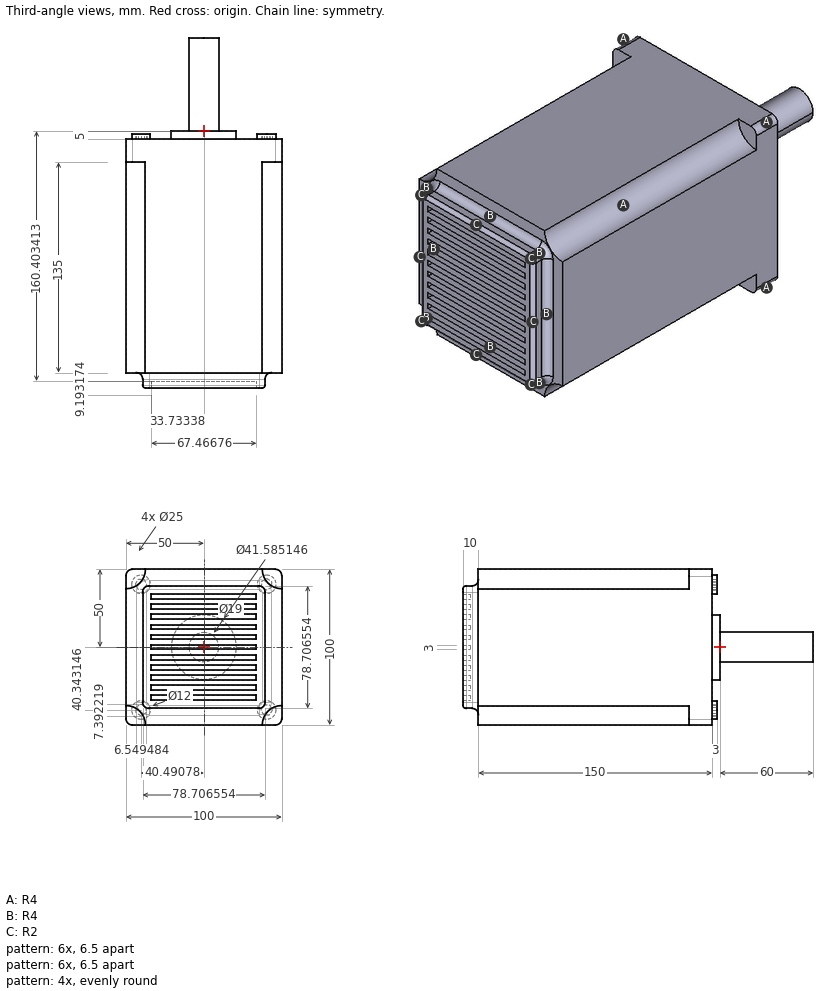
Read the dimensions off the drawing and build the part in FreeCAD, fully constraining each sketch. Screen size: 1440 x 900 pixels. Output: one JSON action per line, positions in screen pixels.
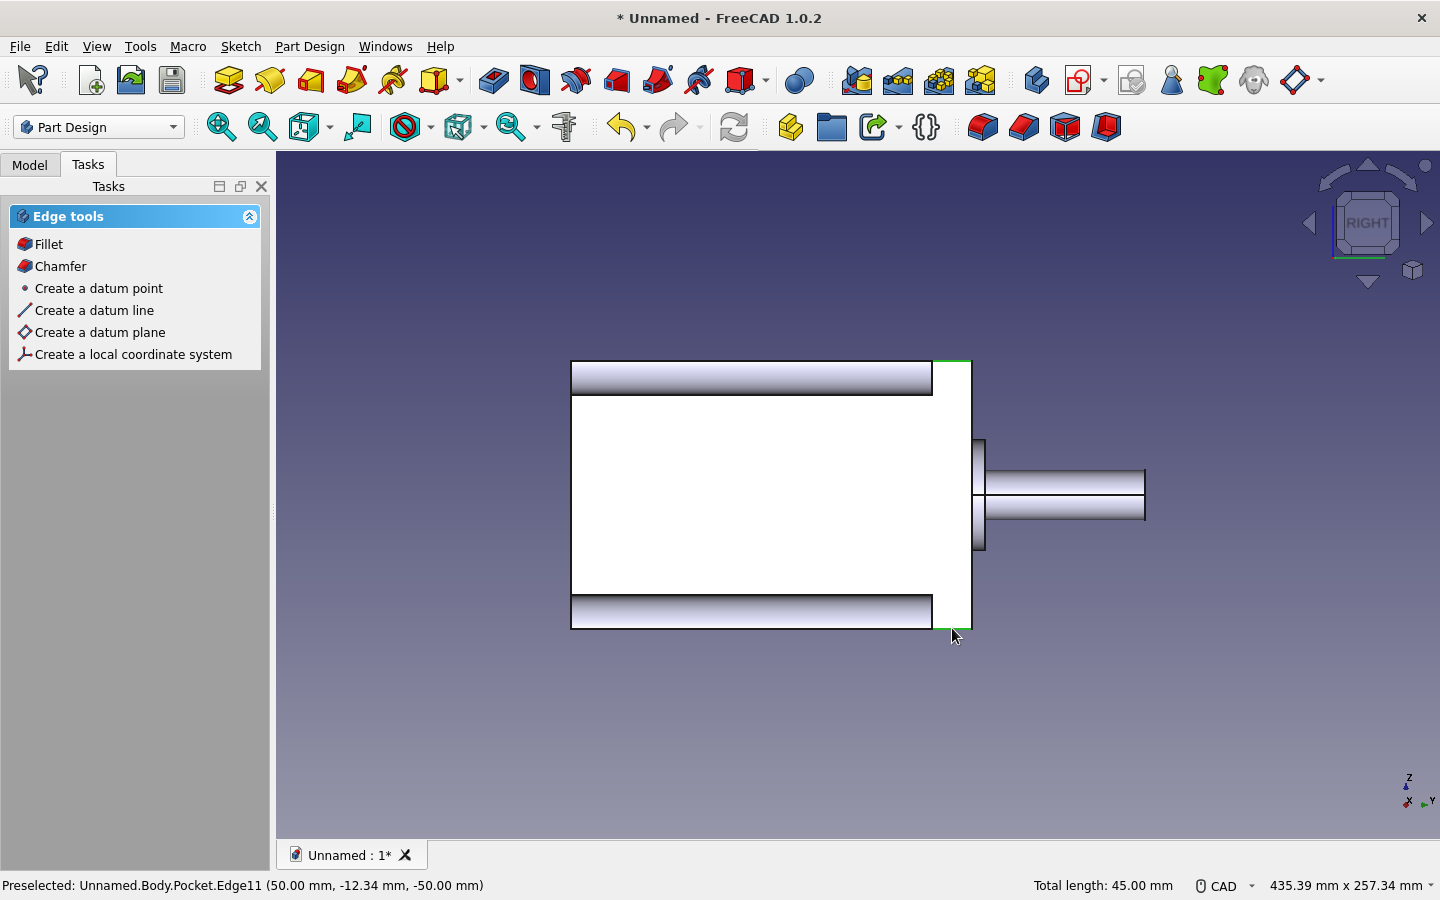
{"action": "key", "text": "5"}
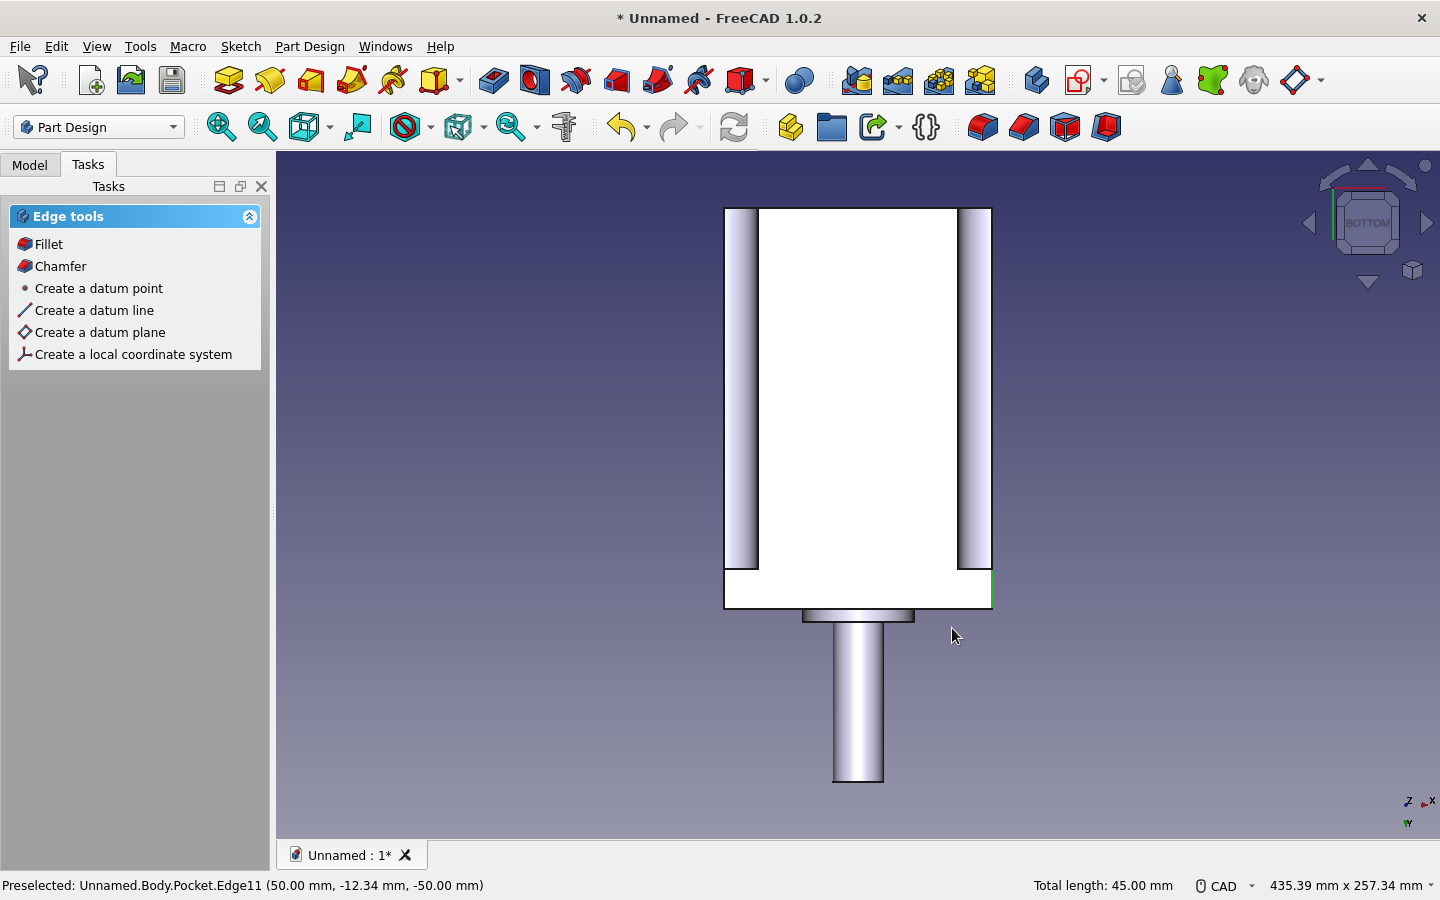
{"action": "left_click", "coordinate": [724, 588], "text": "ctrl"}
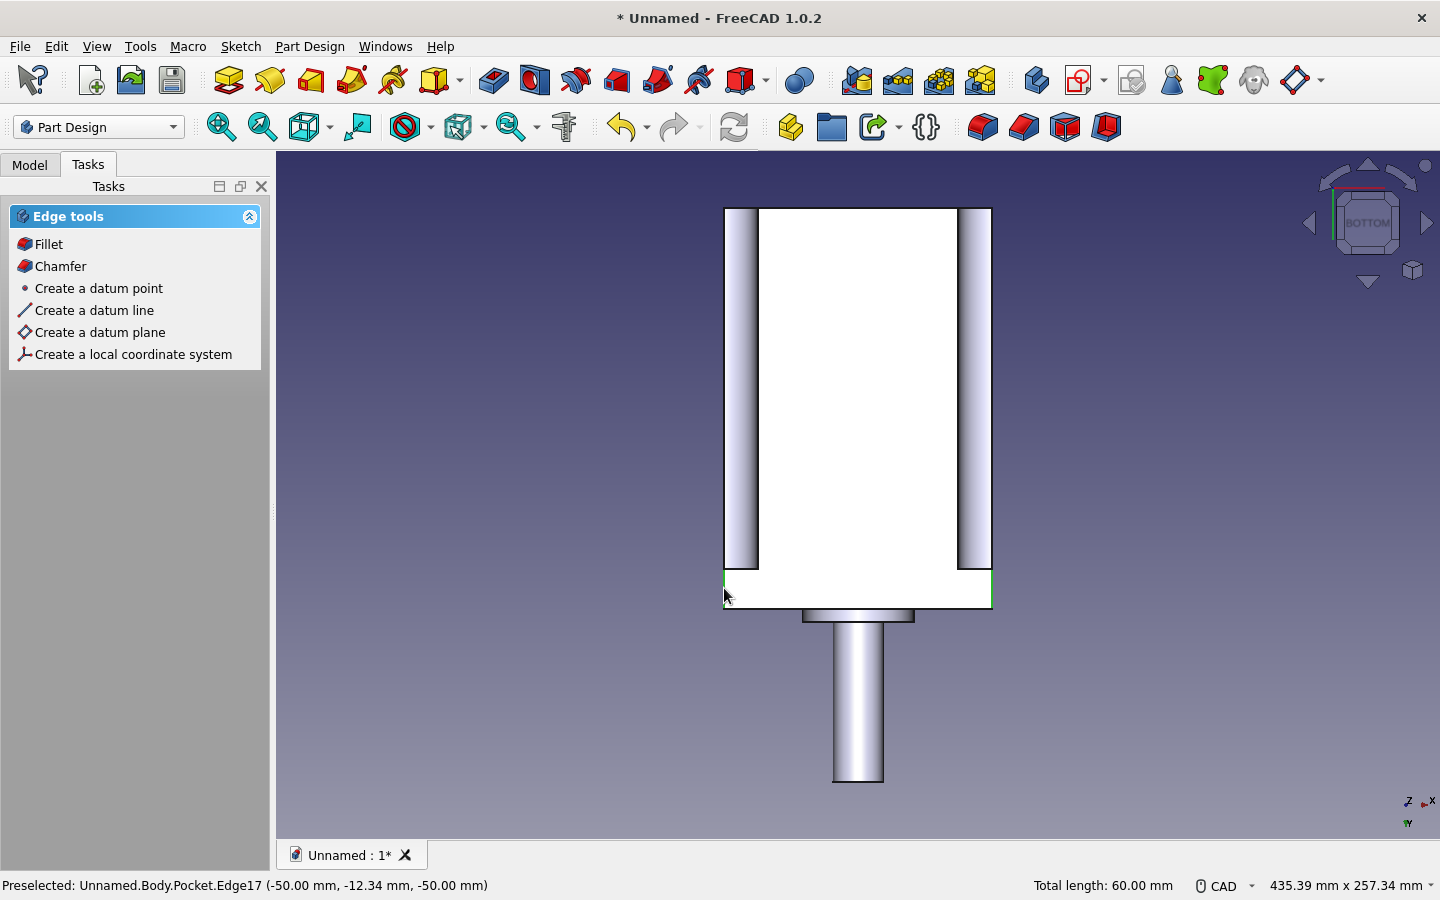
{"action": "left_click", "coordinate": [983, 128]}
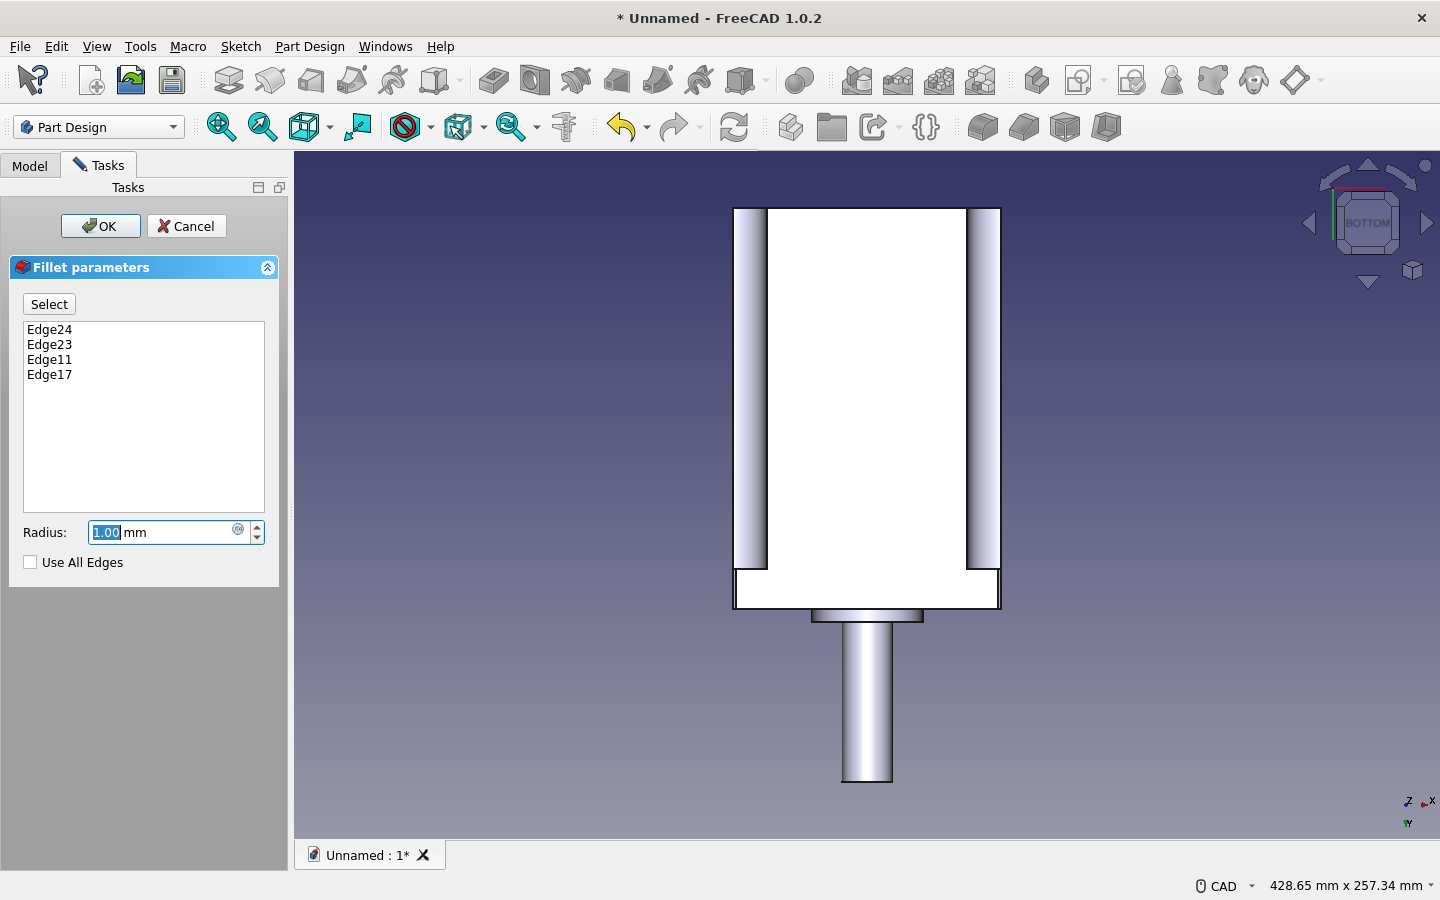
{"action": "type", "text": "4"}
{"action": "key", "text": "Tab"}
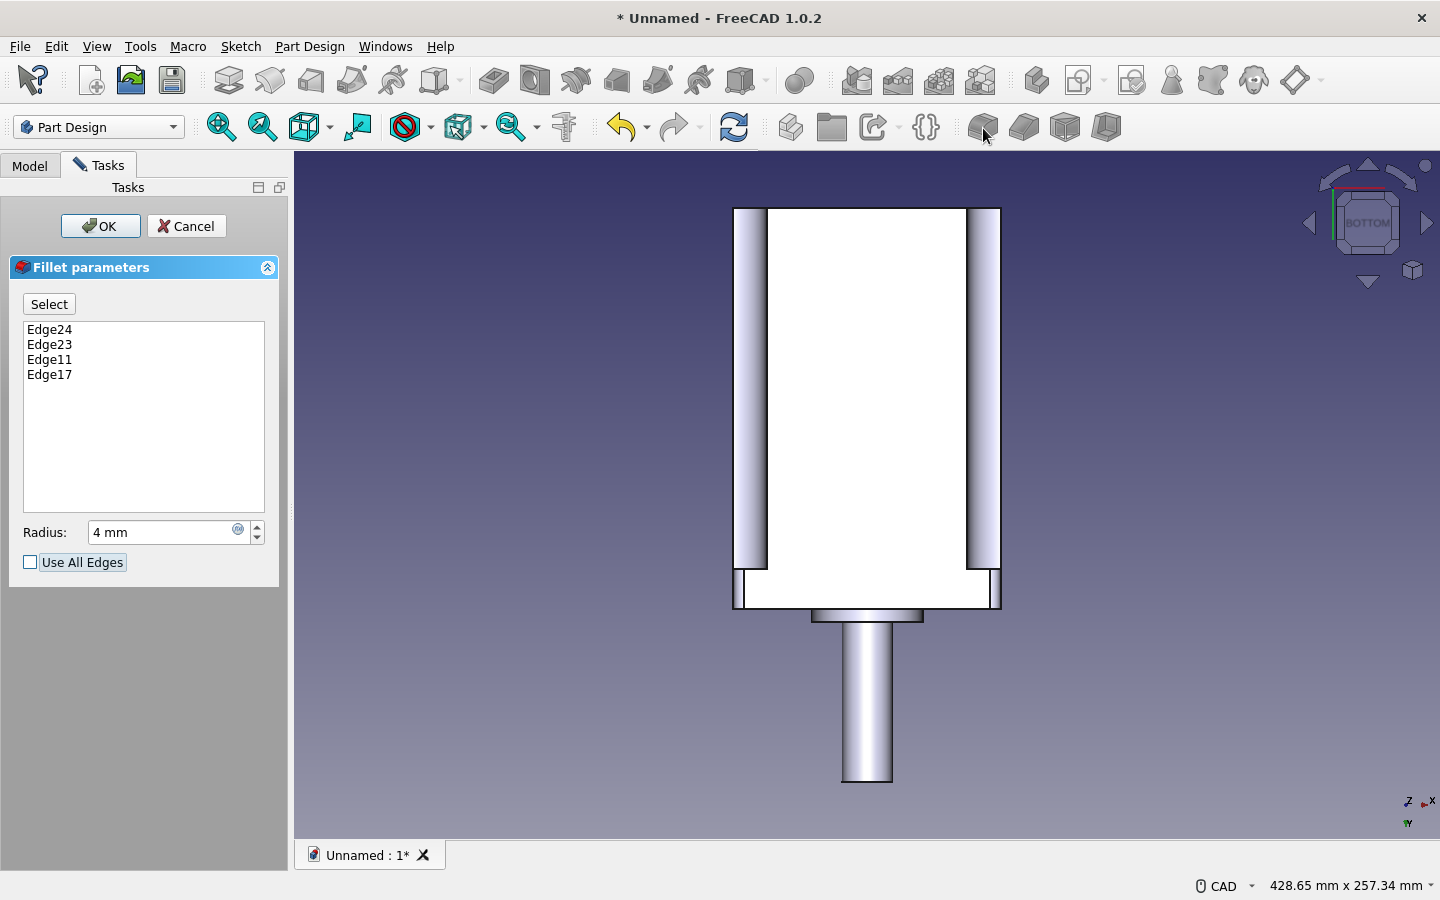
{"action": "left_click", "coordinate": [101, 226]}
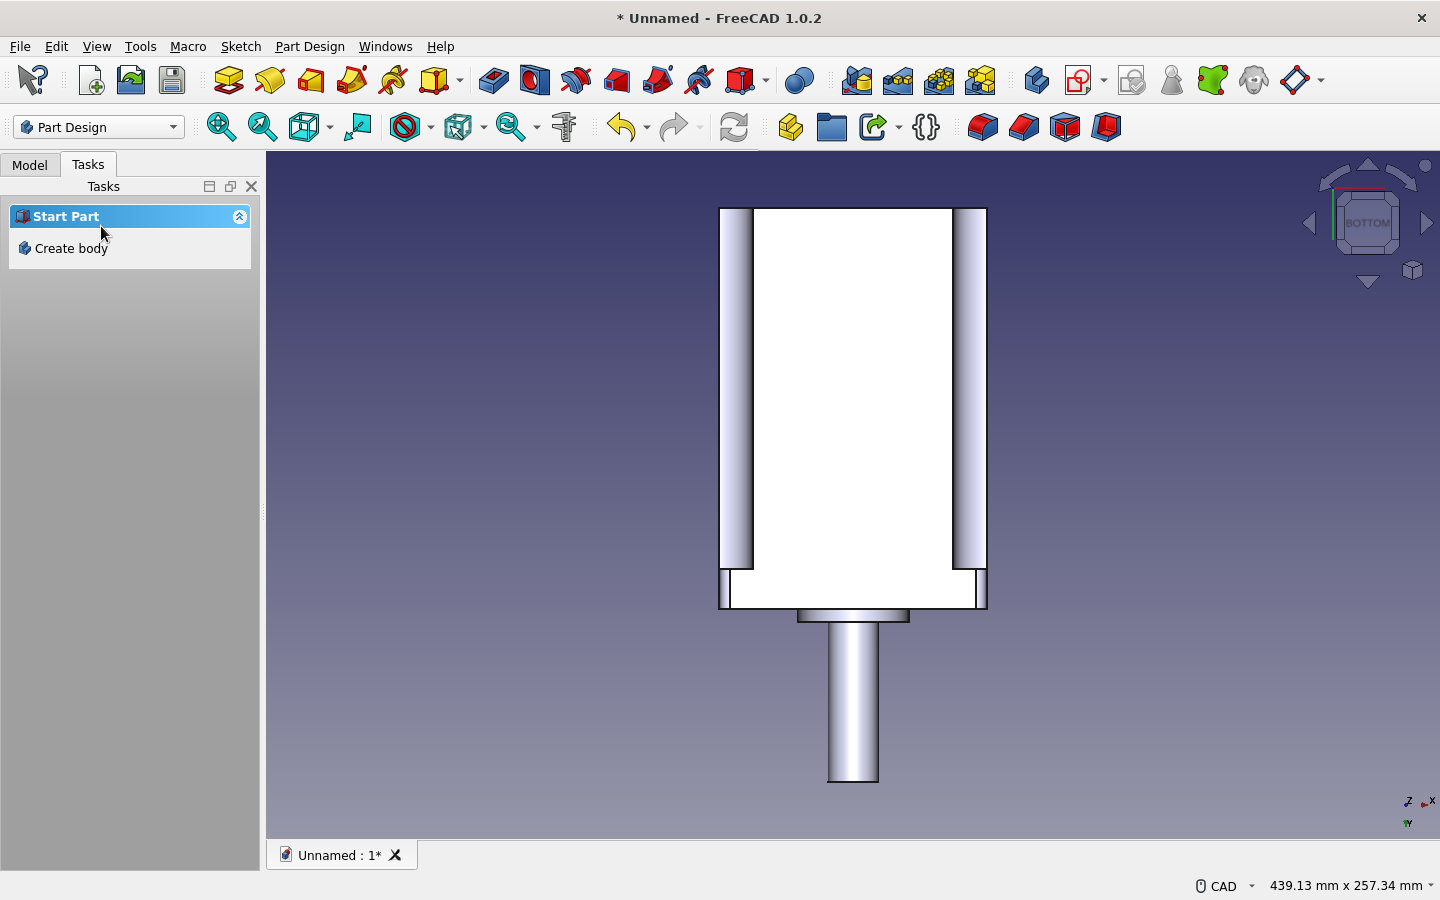
{"action": "key", "text": "0"}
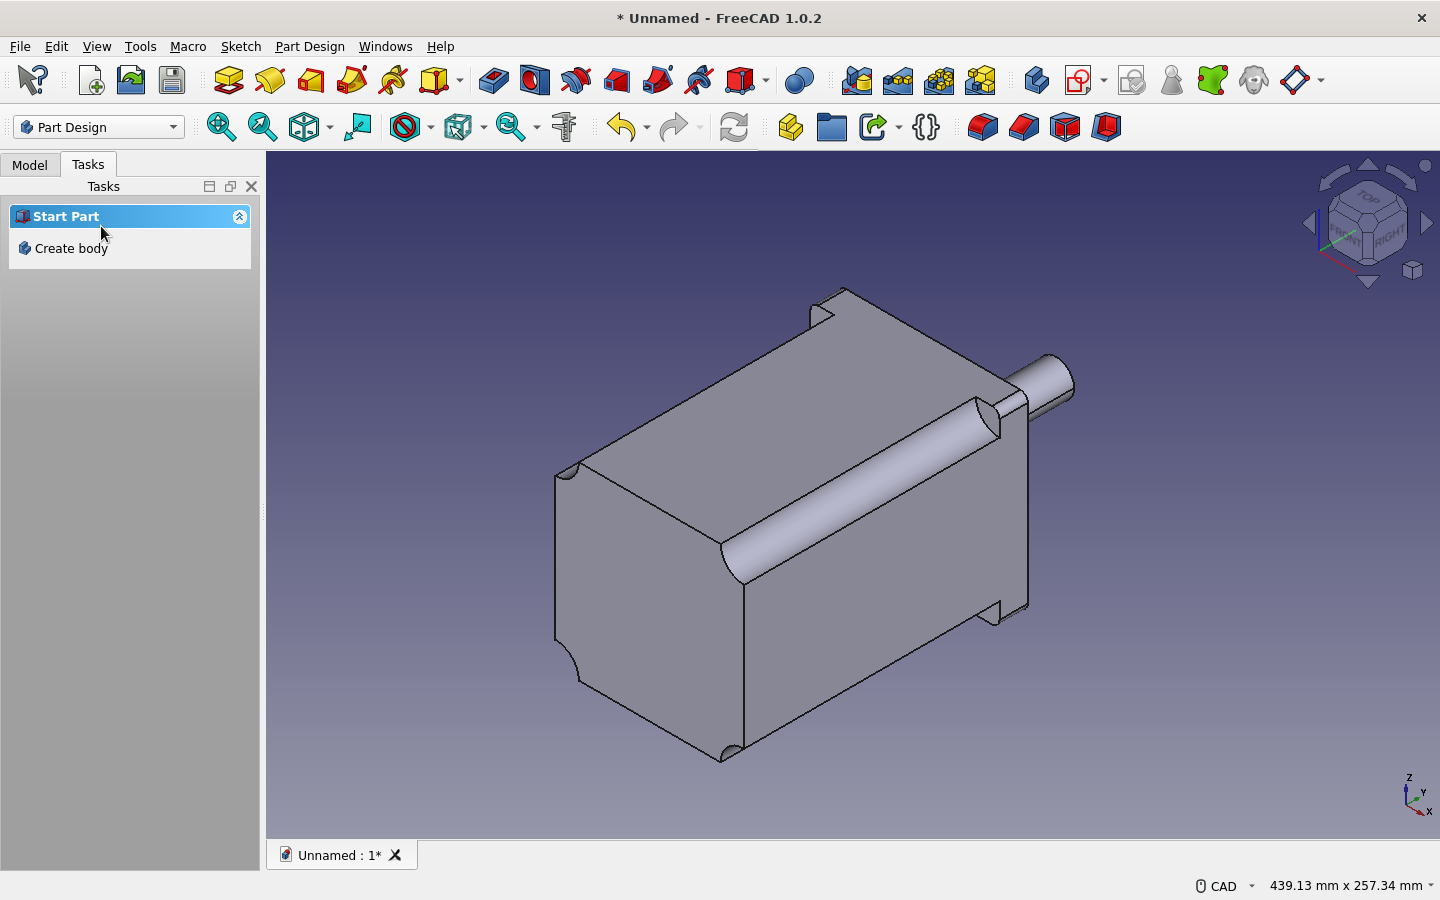
{"action": "left_click", "coordinate": [650, 611]}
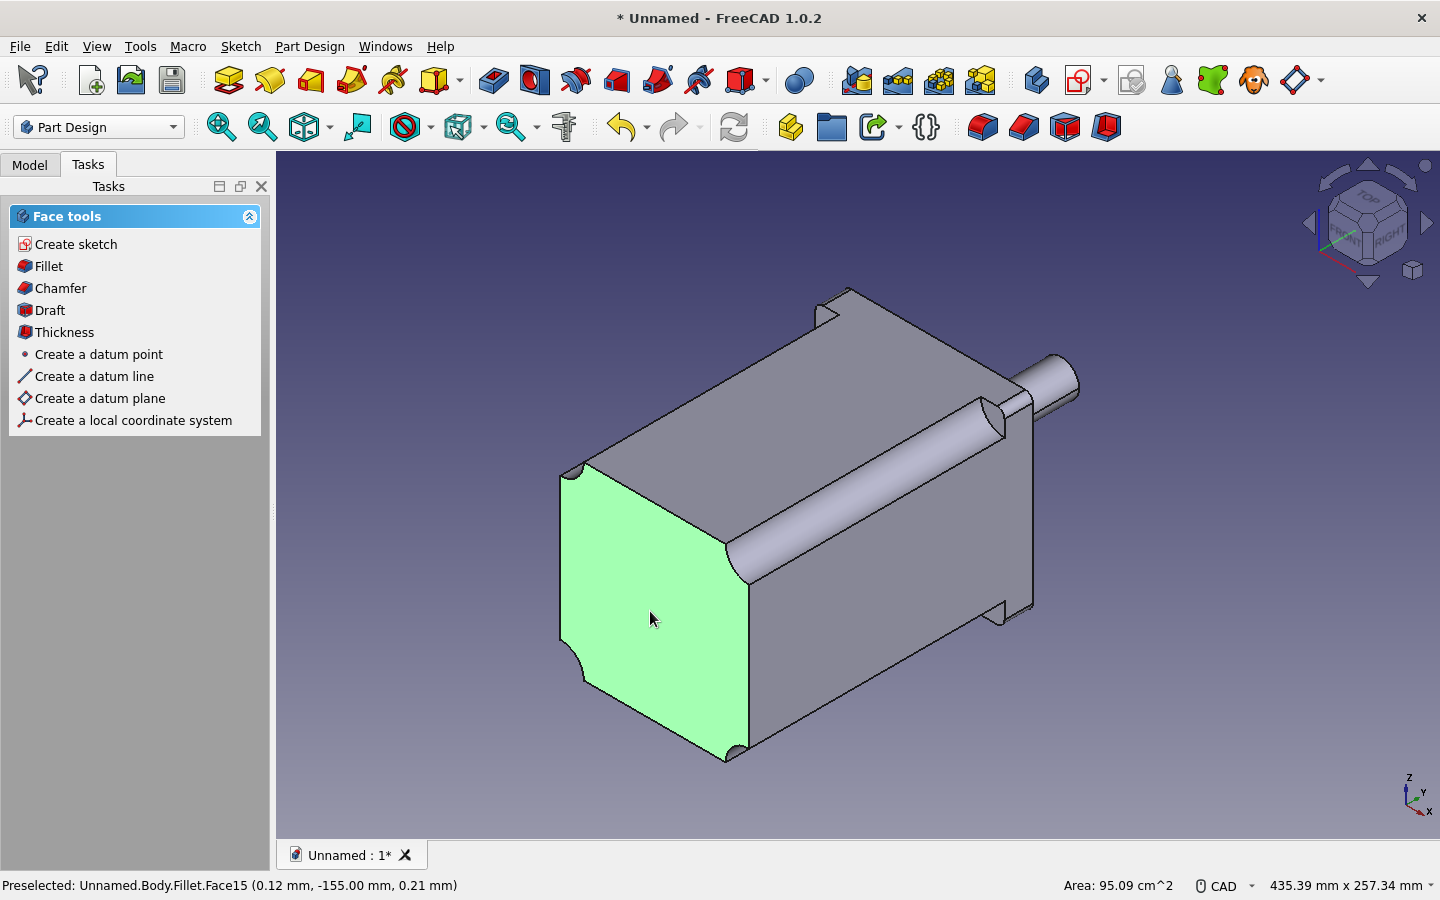
{"action": "left_click", "coordinate": [1078, 80]}